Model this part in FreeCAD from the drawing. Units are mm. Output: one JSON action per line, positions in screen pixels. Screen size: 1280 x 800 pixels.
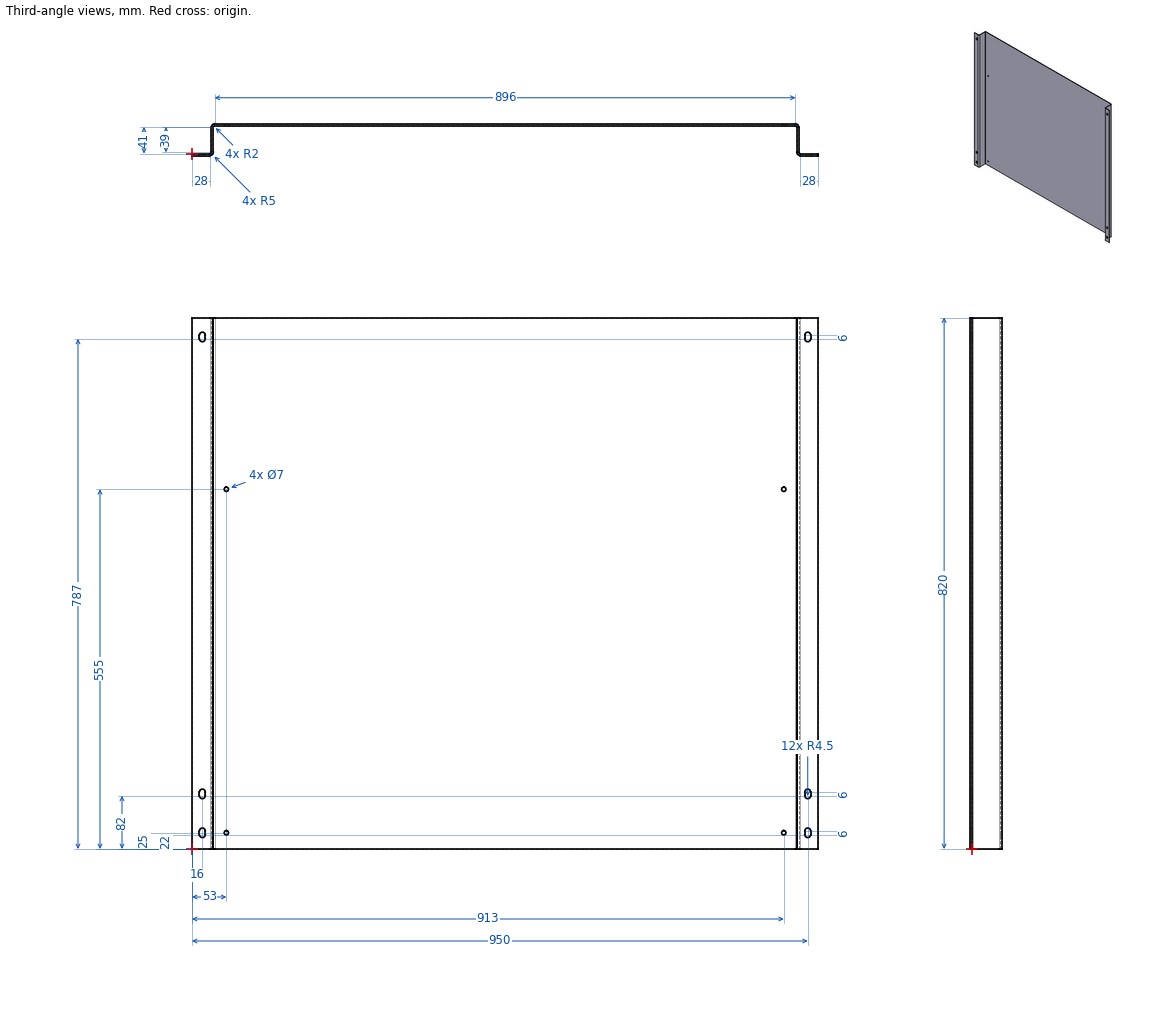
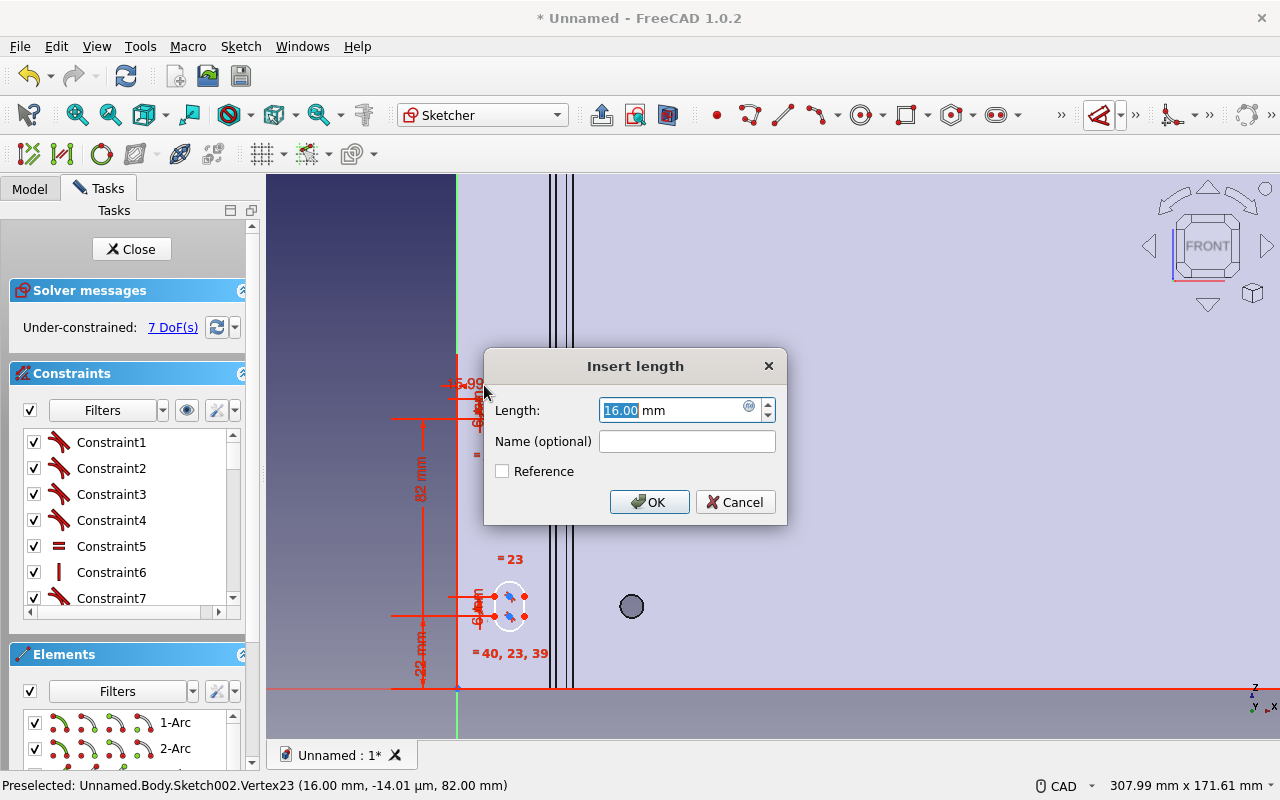
{"action": "type", "text": "16"}
{"action": "key", "text": "Return"}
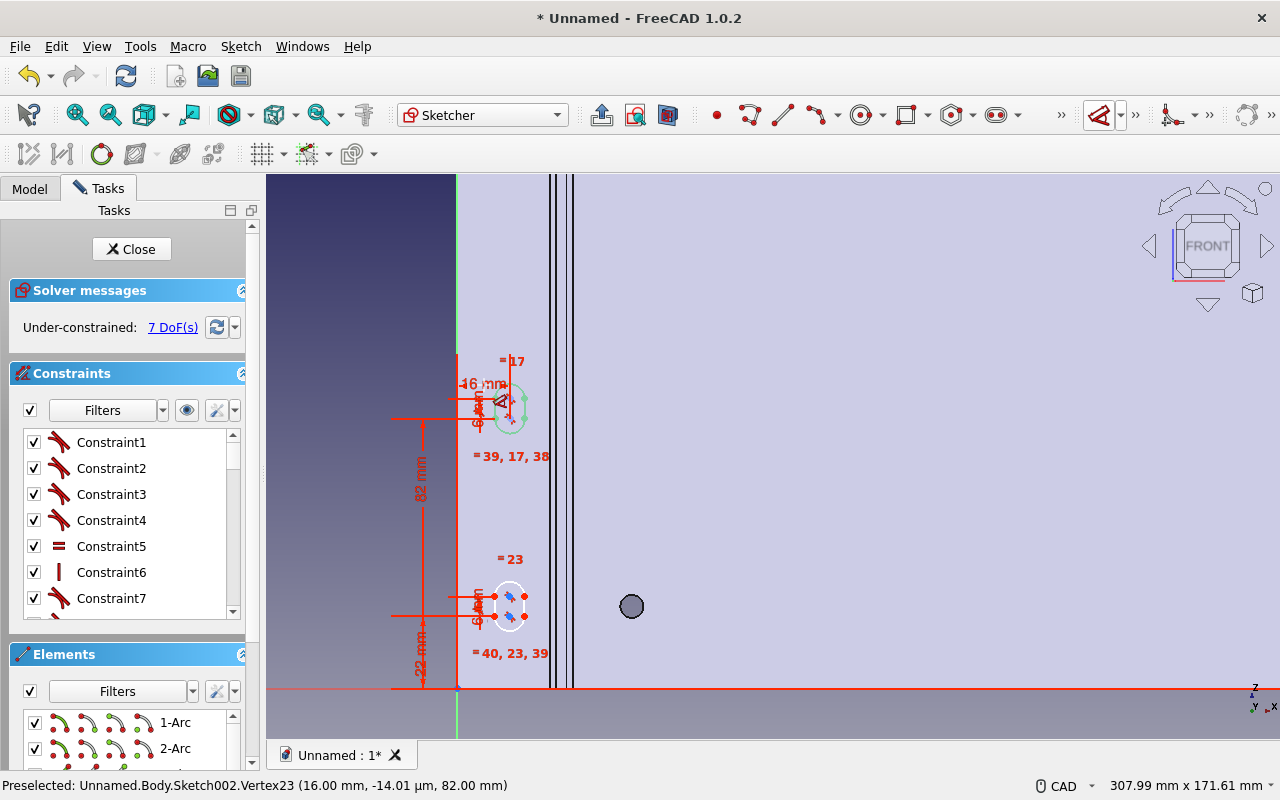
{"action": "left_click", "coordinate": [510, 616]}
{"action": "left_click", "coordinate": [483, 582]}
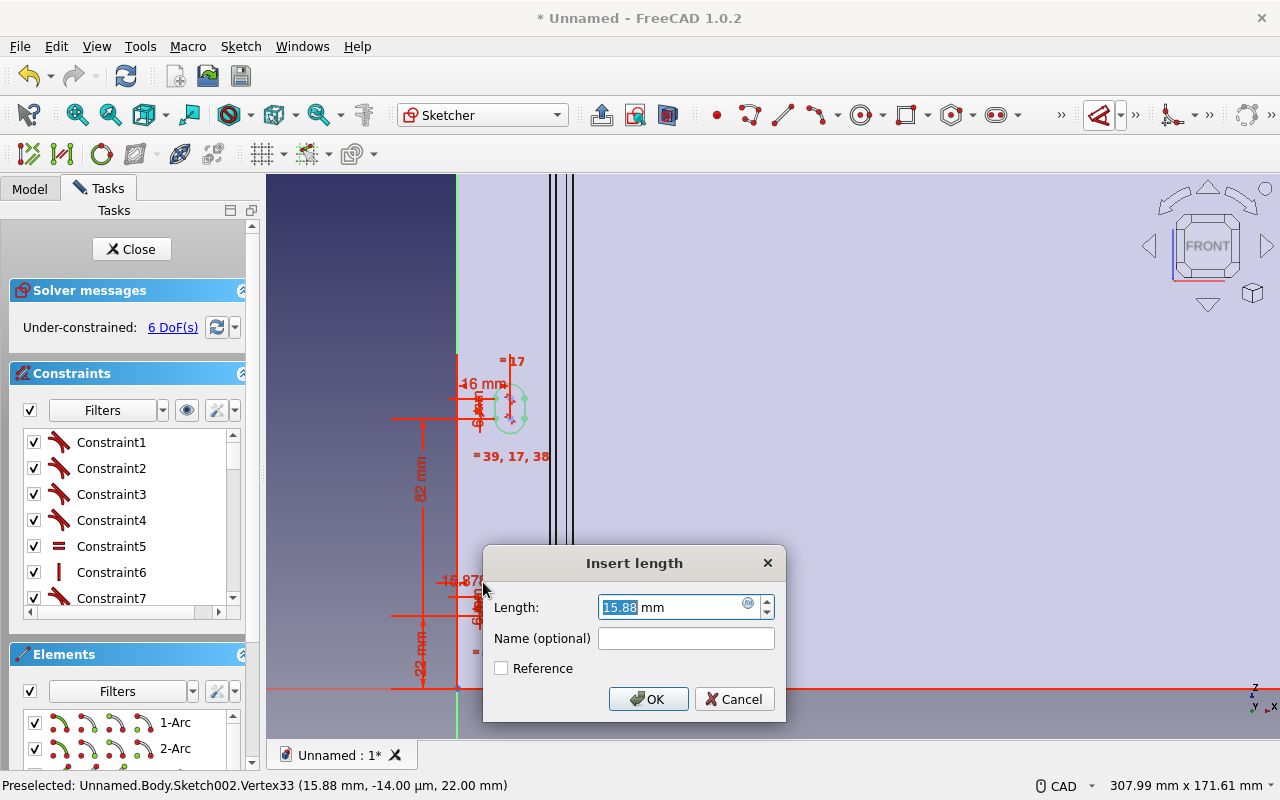
{"action": "type", "text": "16"}
{"action": "key", "text": "Return"}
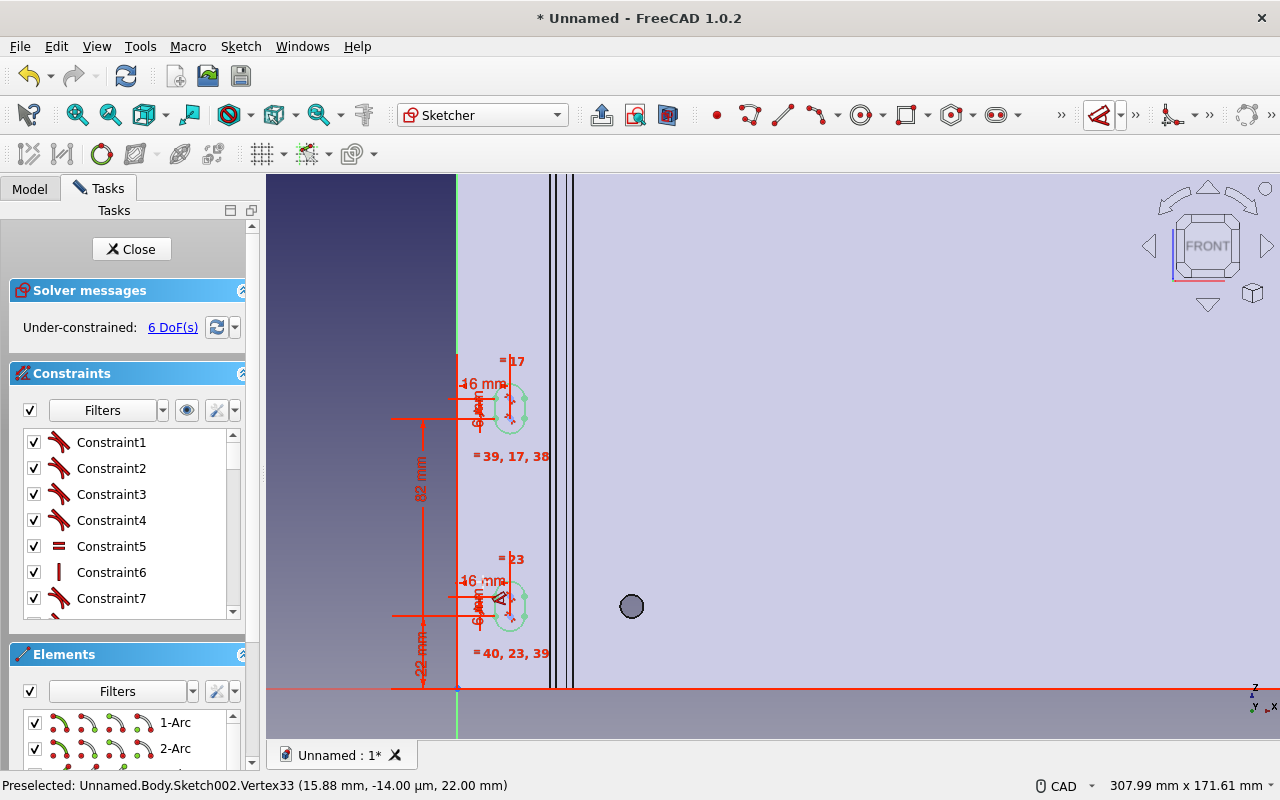
{"action": "scroll", "coordinate": [497, 626], "scroll_direction": "down", "scroll_amount": 10}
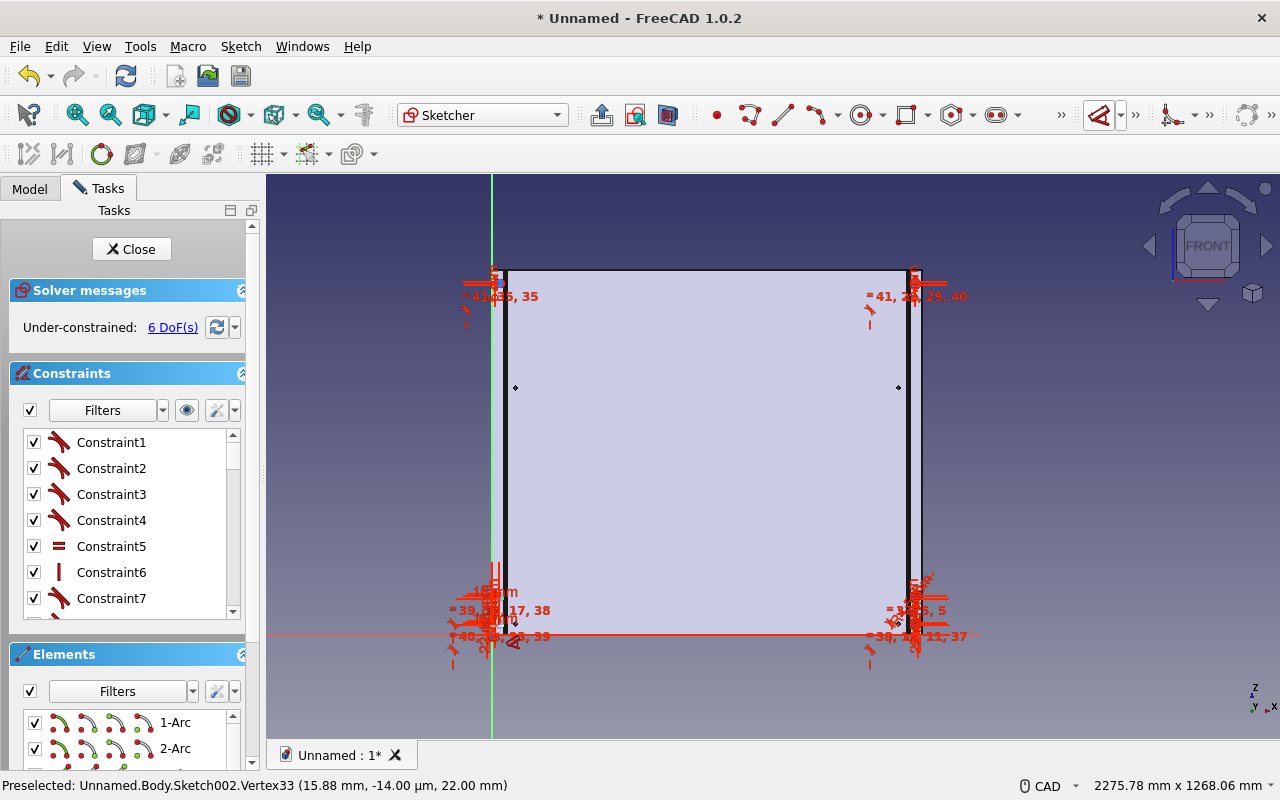
{"action": "scroll", "coordinate": [499, 285], "scroll_direction": "up", "scroll_amount": 10}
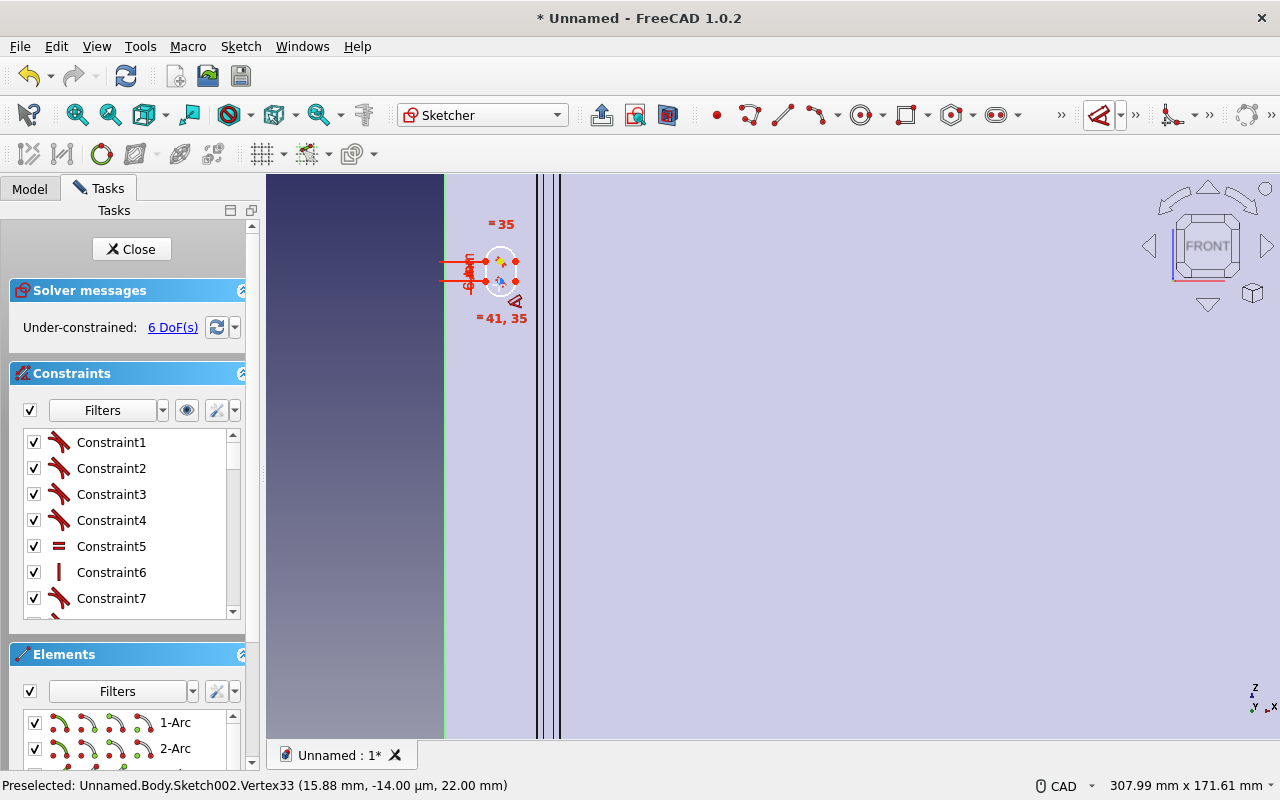
{"action": "left_click", "coordinate": [501, 281]}
{"action": "left_click", "coordinate": [473, 247]}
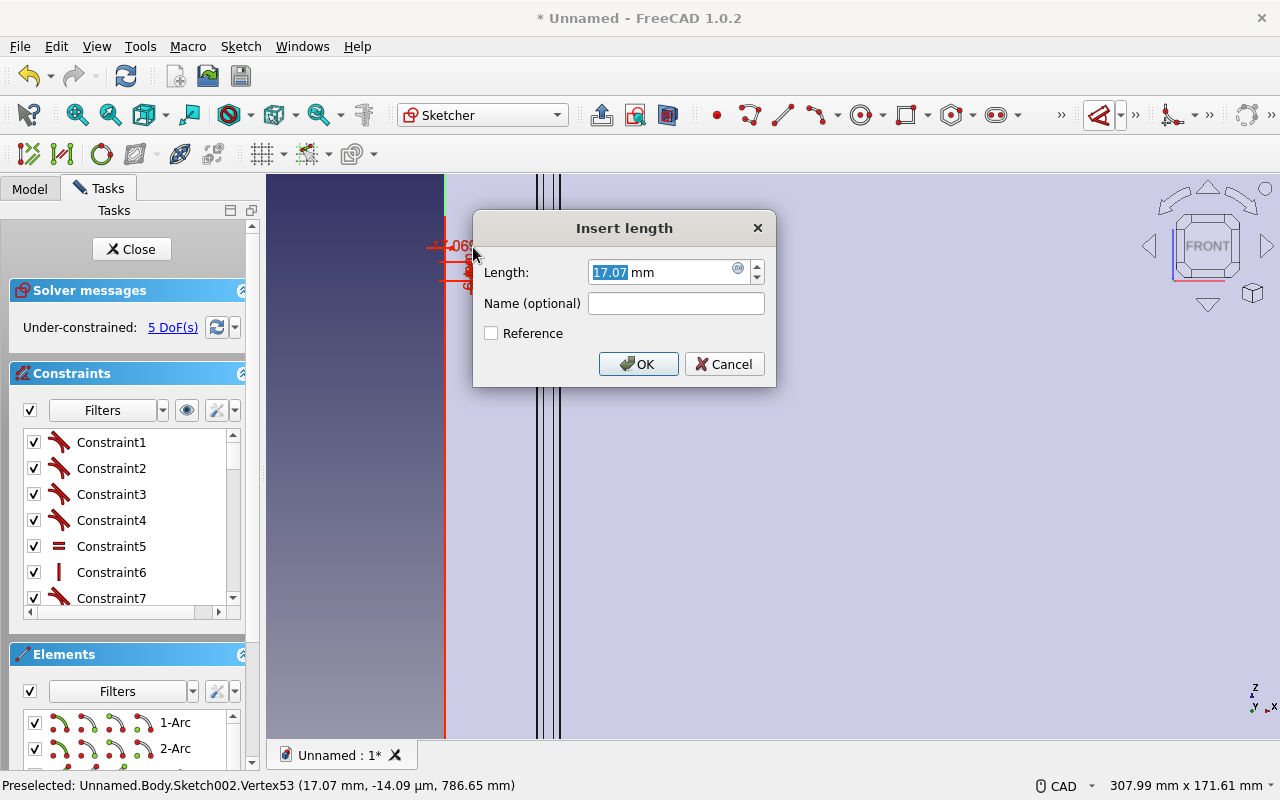
{"action": "type", "text": "16"}
{"action": "key", "text": "Return"}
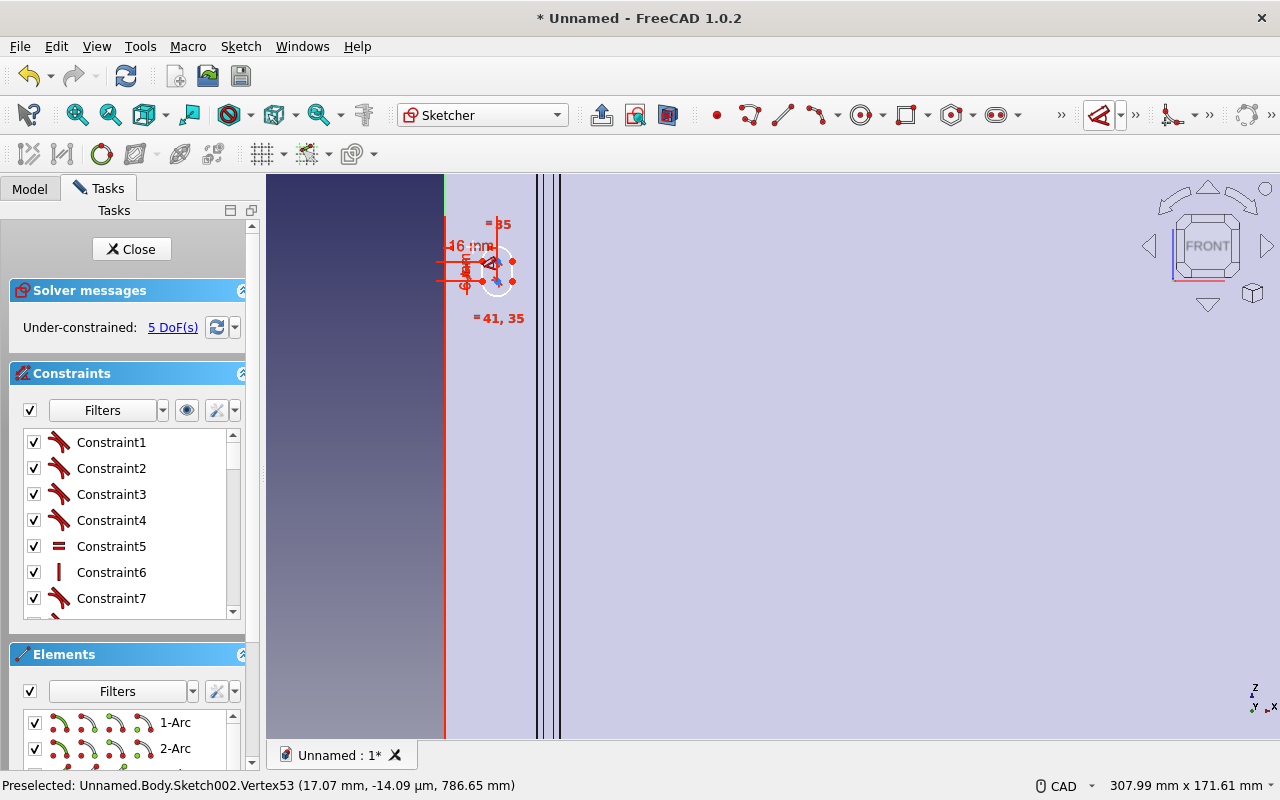
{"action": "scroll", "coordinate": [499, 284], "scroll_direction": "down", "scroll_amount": 10}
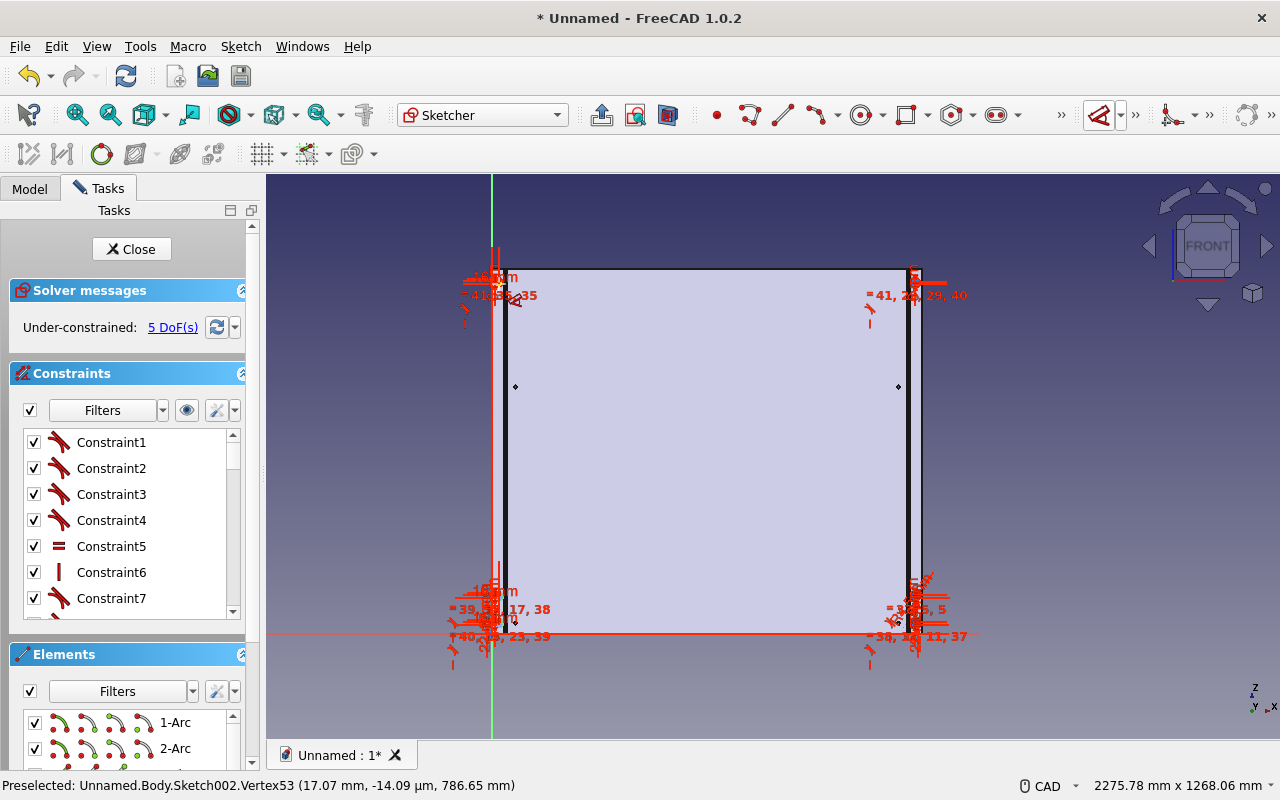
{"action": "scroll", "coordinate": [913, 284], "scroll_direction": "up", "scroll_amount": 10}